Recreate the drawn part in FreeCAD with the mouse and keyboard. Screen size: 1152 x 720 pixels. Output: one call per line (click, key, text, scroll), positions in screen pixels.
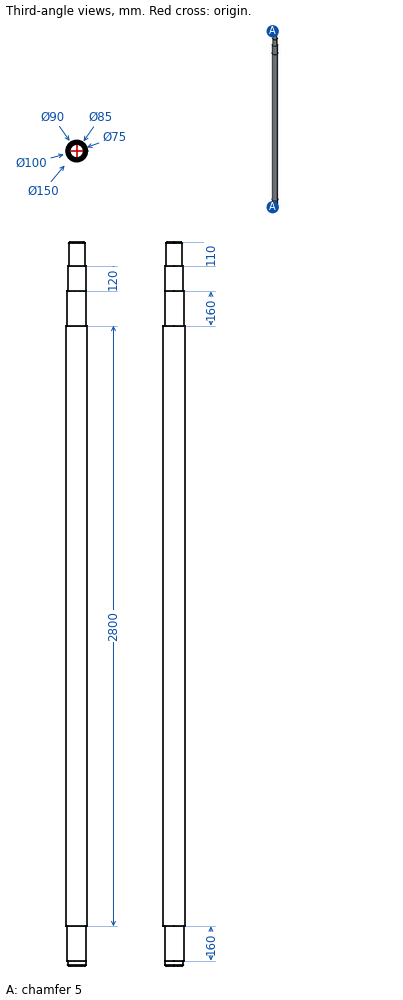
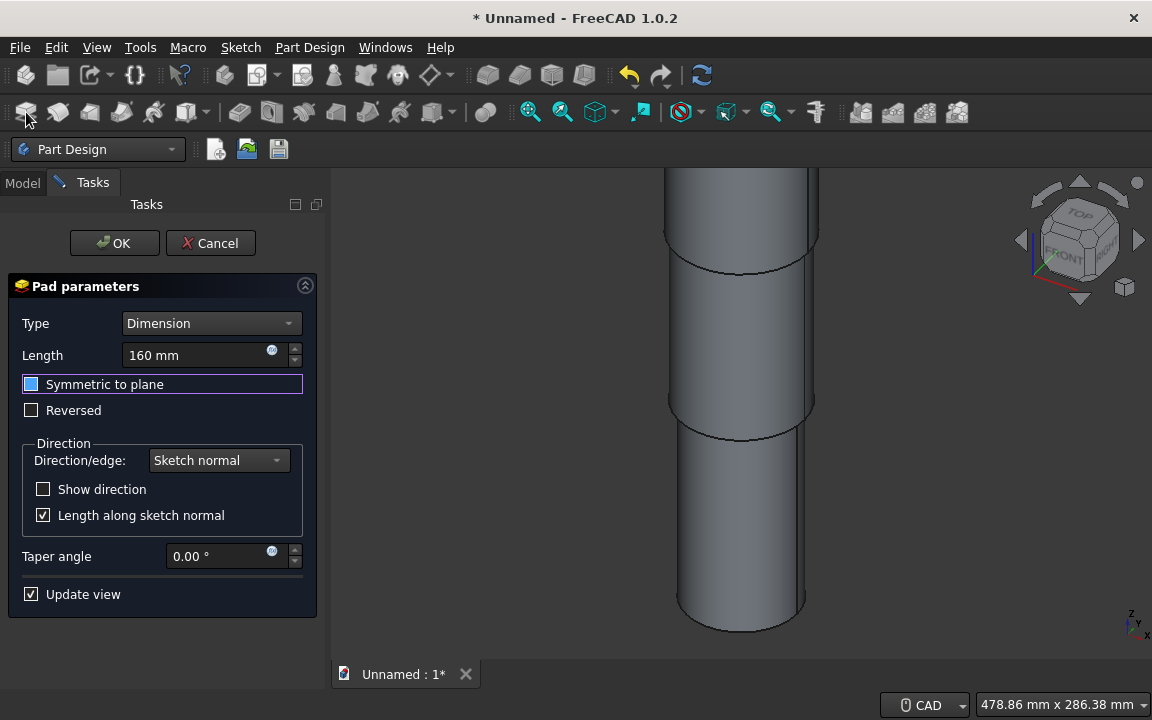
click(115, 243)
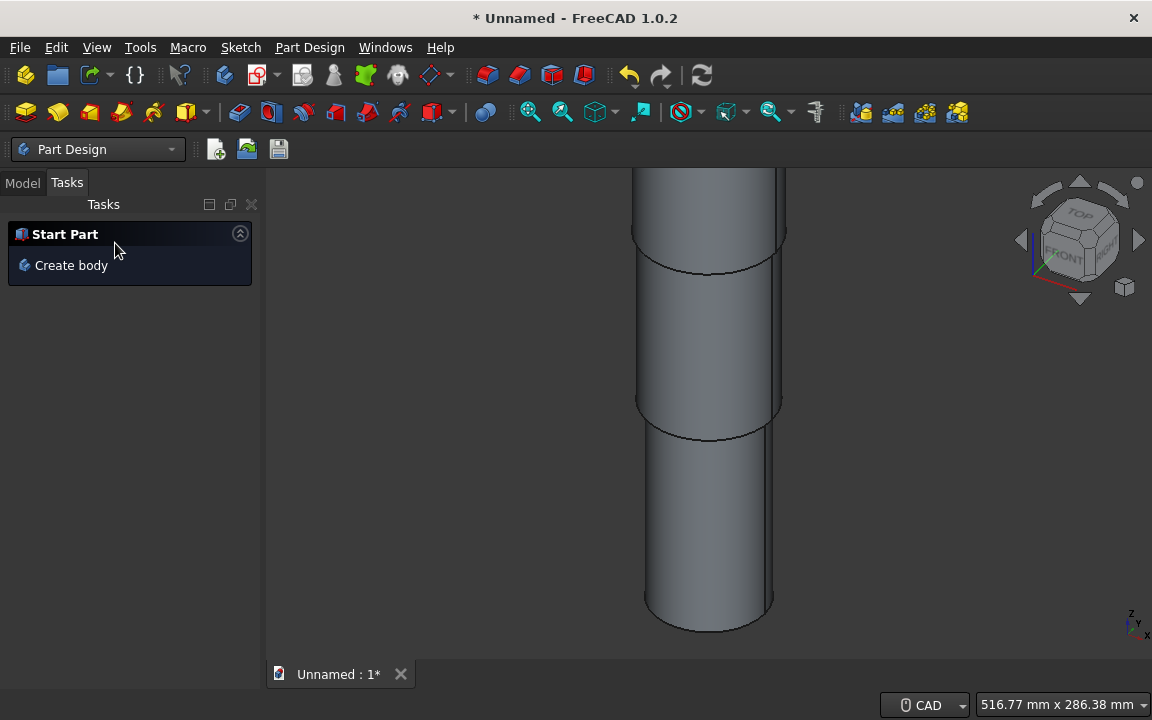
click(532, 112)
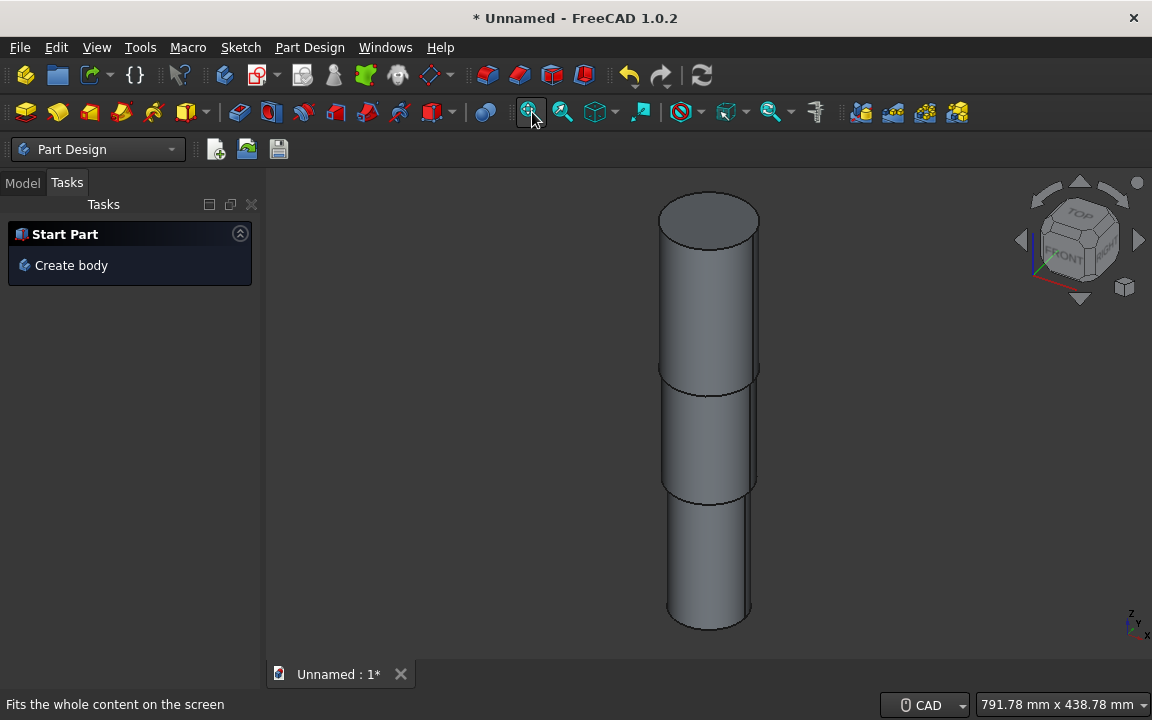
click(709, 220)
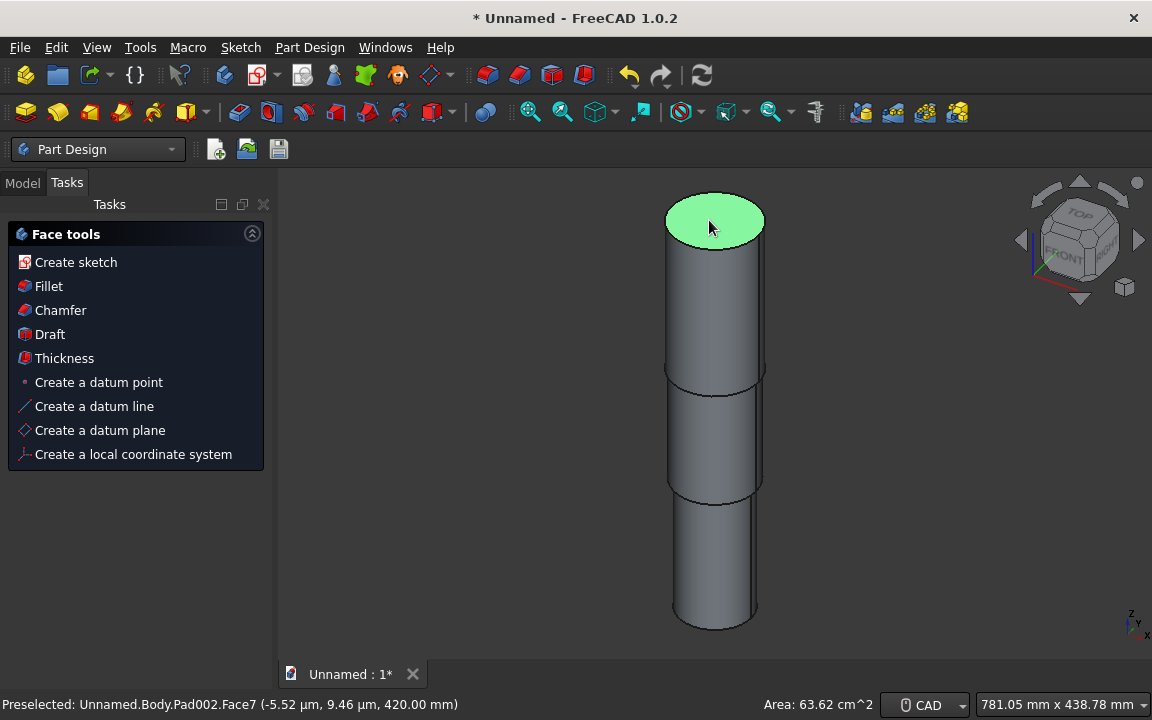
click(258, 76)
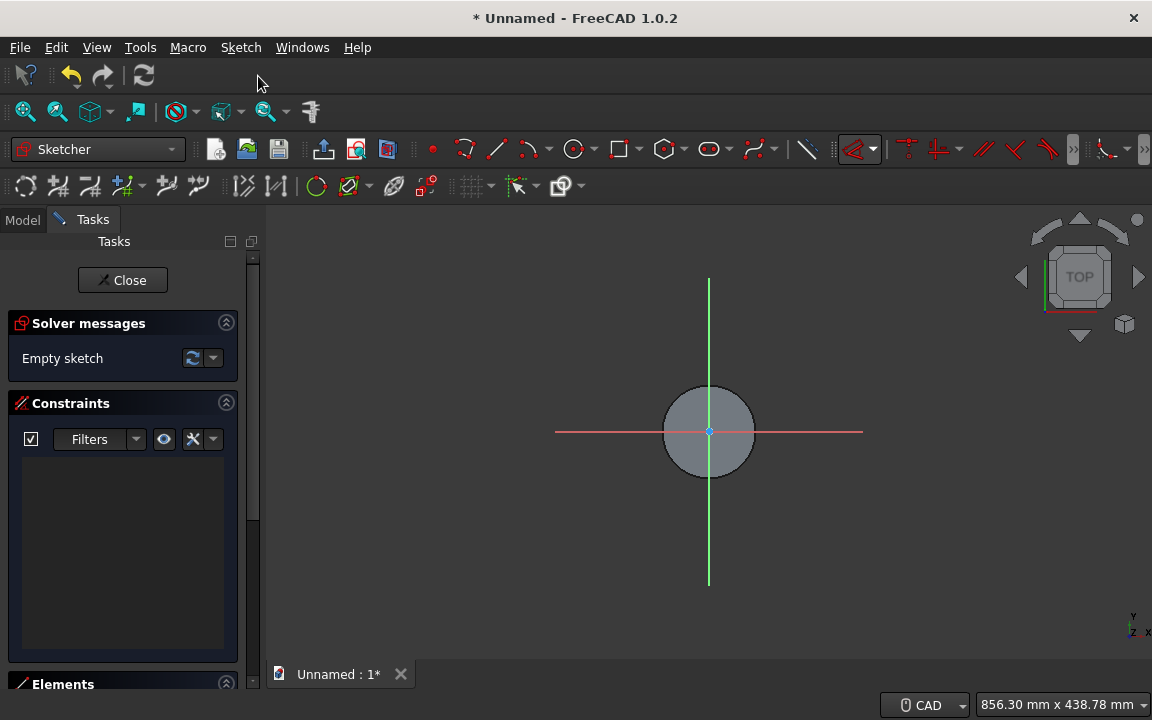
scroll(749, 432, up, 5)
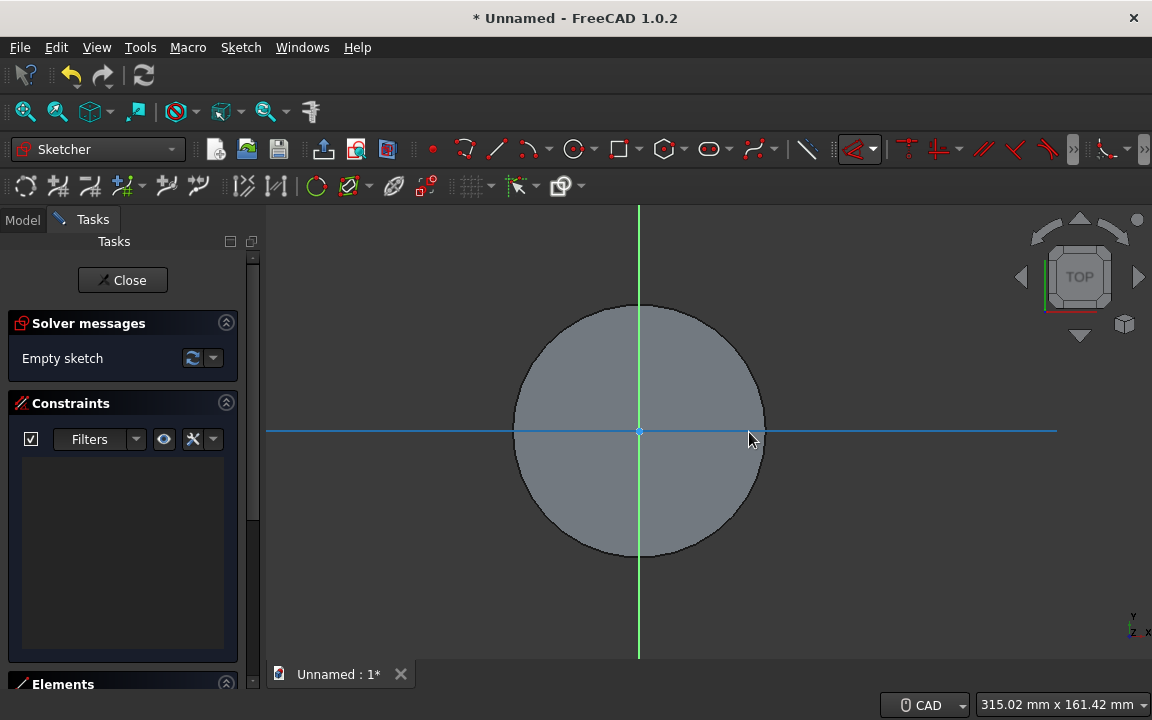
click(574, 150)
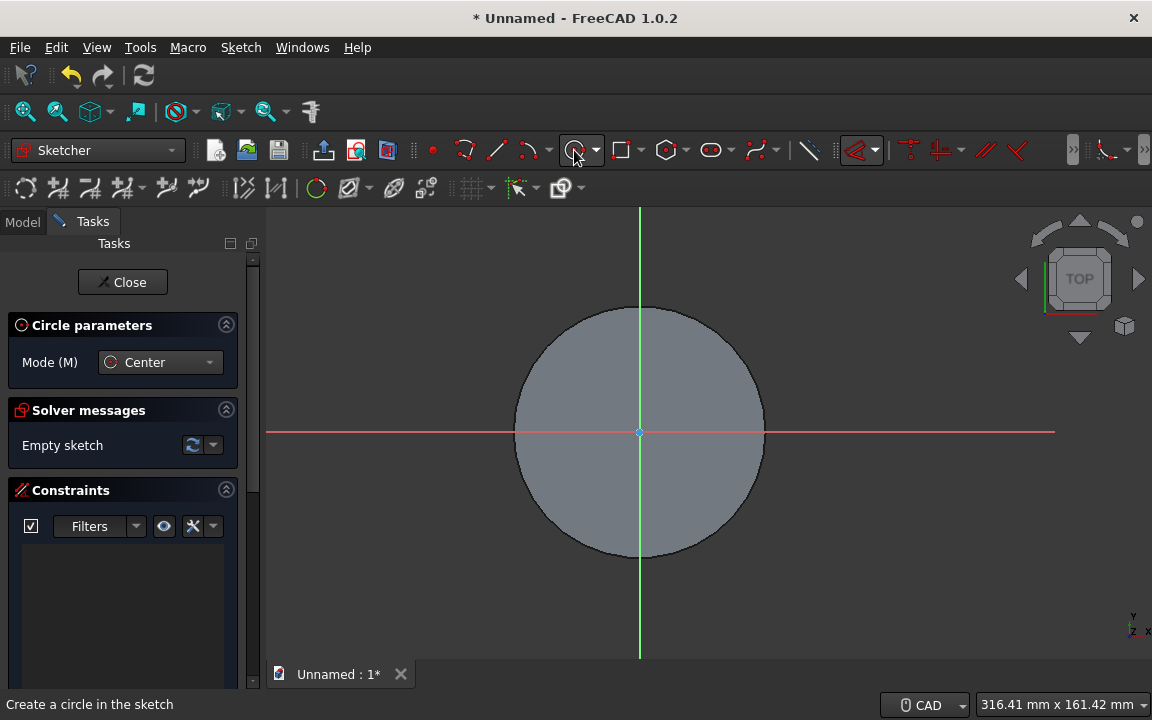
click(640, 432)
click(739, 333)
key(Escape)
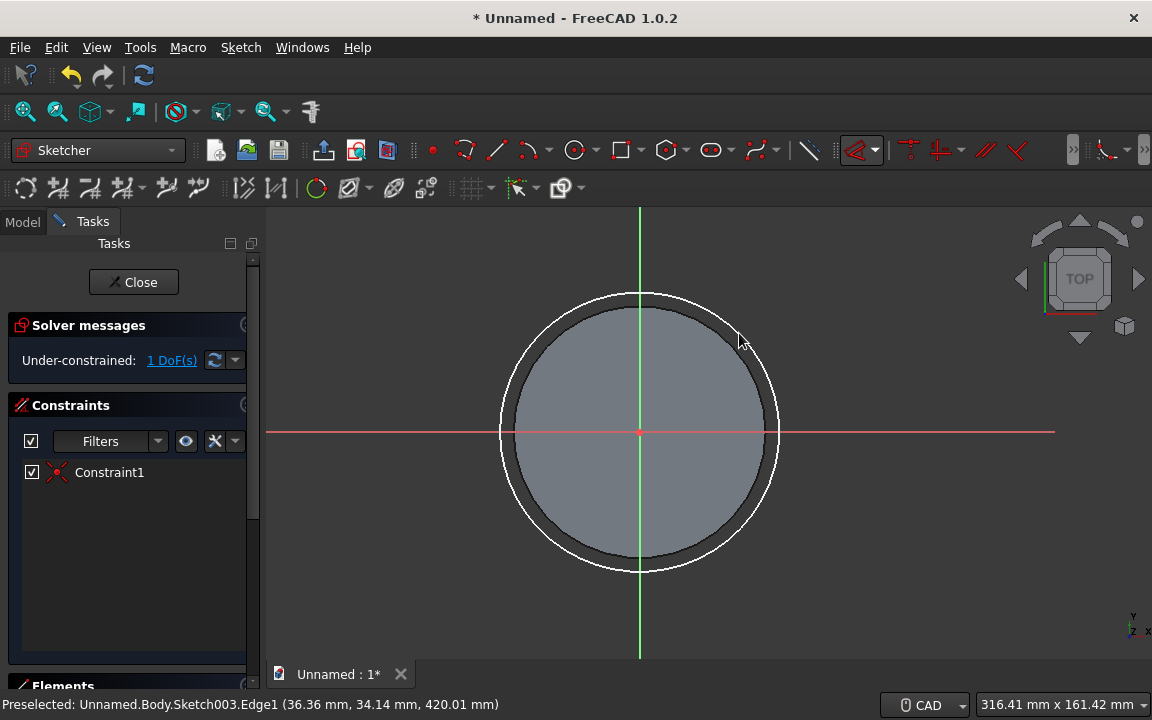
click(738, 333)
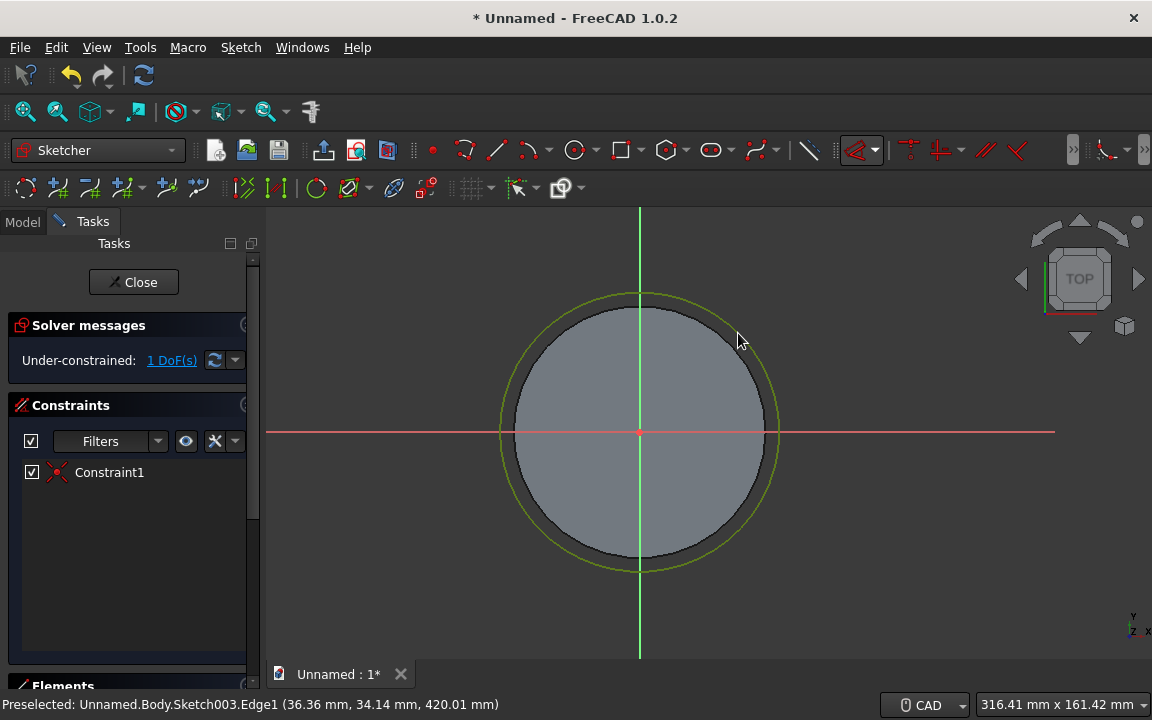
click(878, 150)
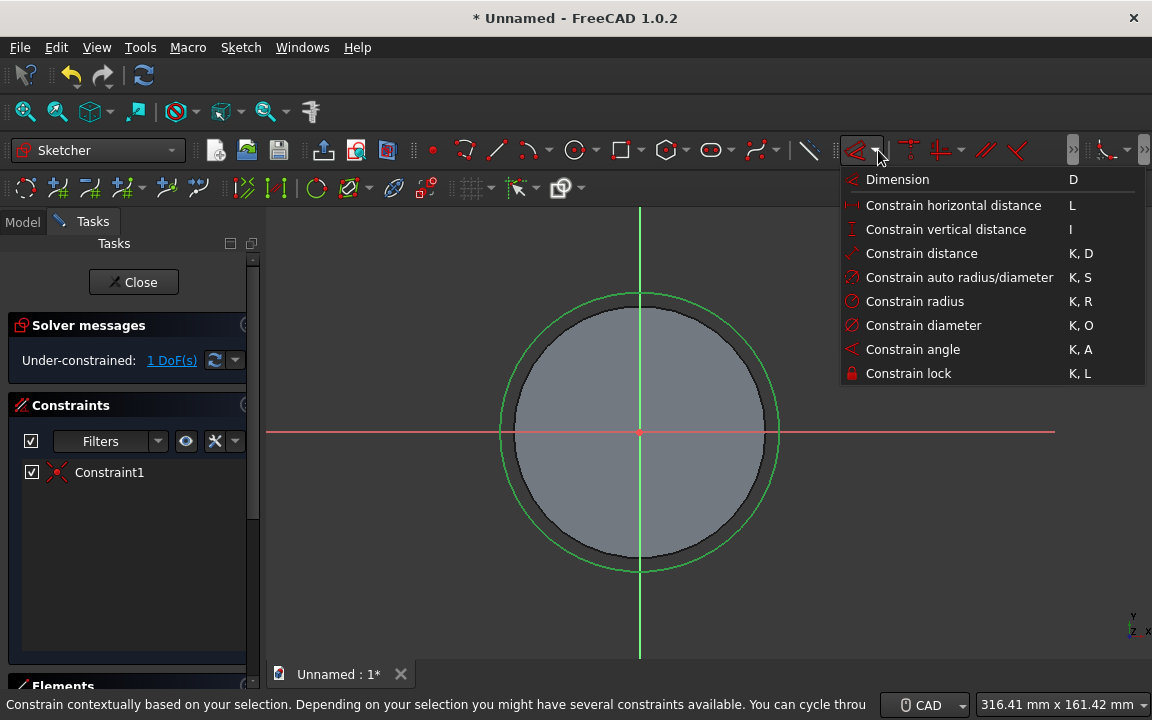
click(993, 325)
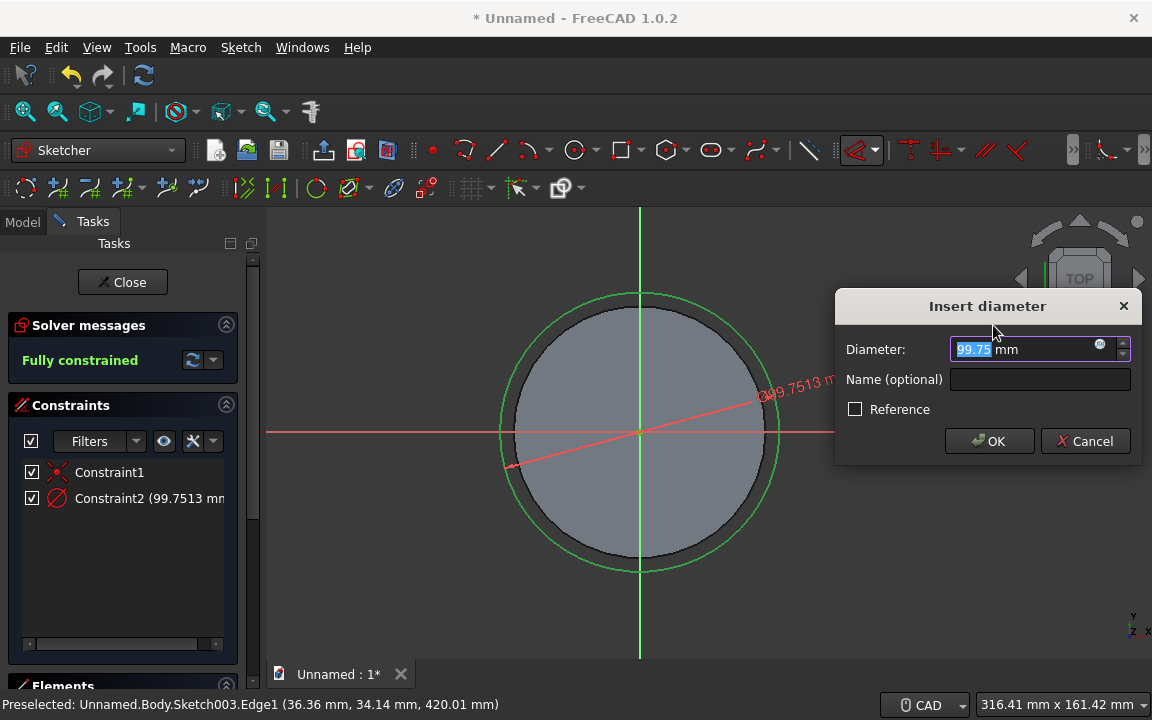
text(100)
key(Return)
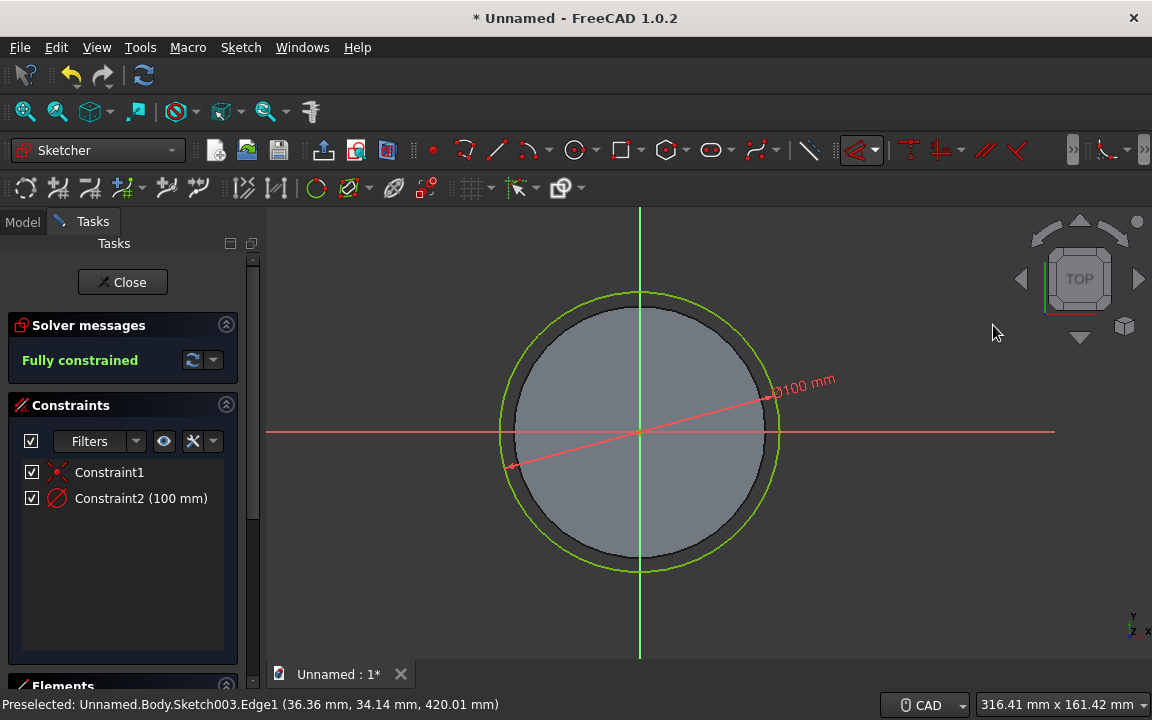
click(123, 282)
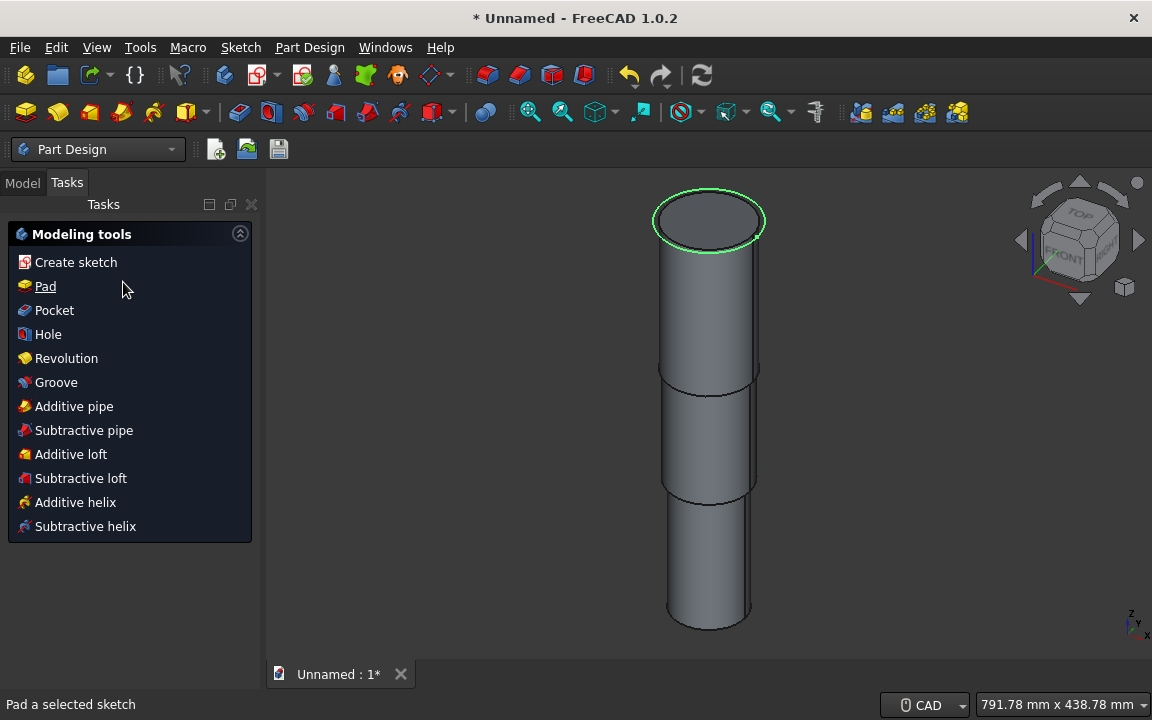
click(26, 112)